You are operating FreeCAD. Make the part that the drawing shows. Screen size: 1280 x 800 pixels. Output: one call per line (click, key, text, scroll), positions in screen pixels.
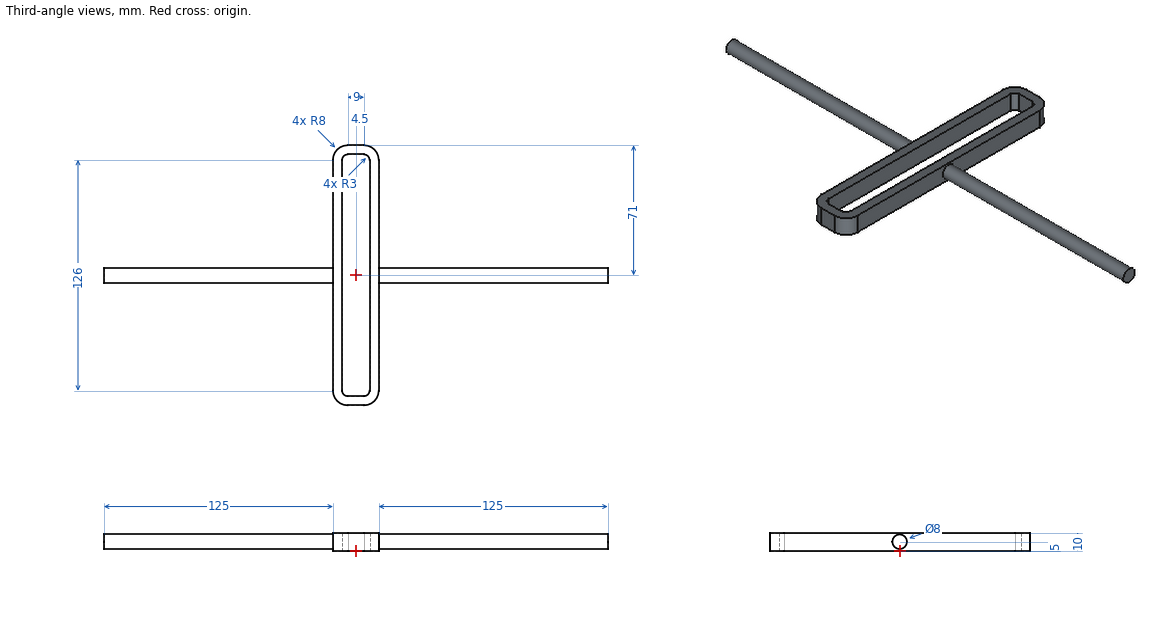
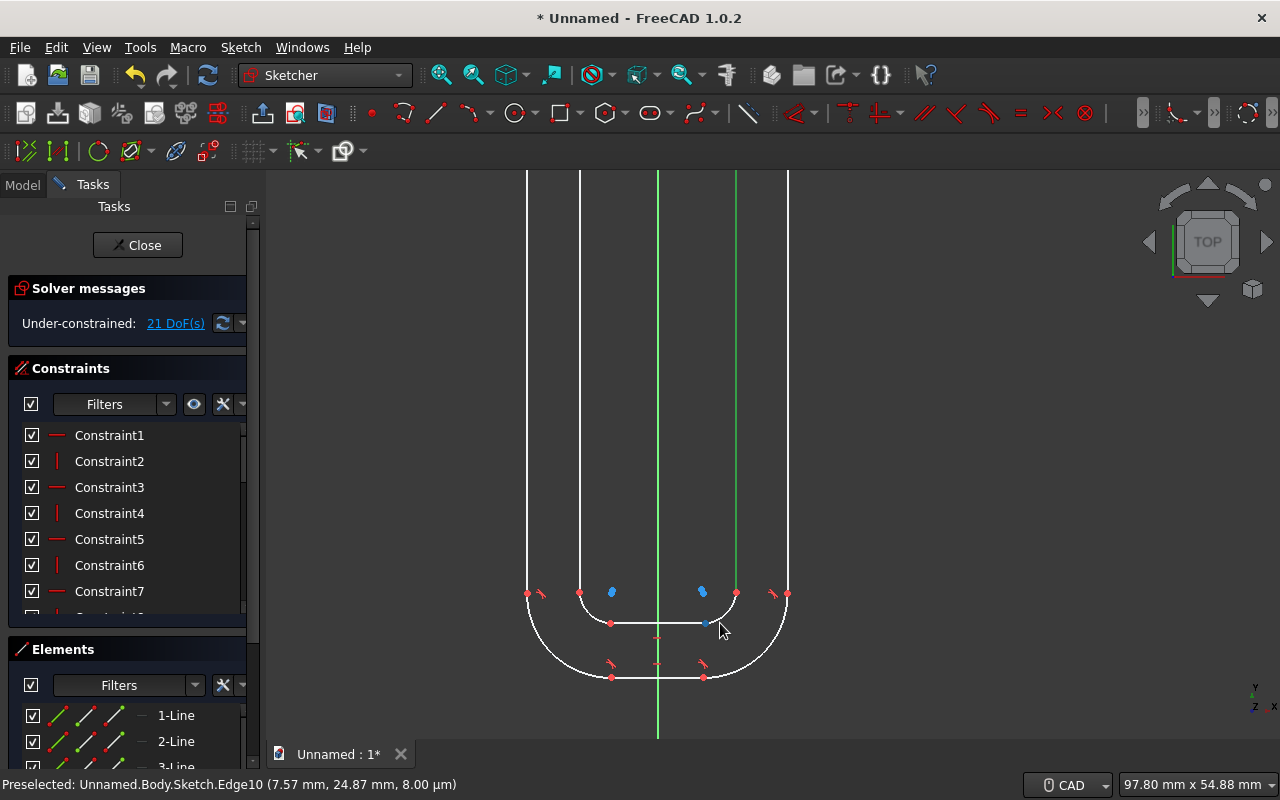
click(719, 619)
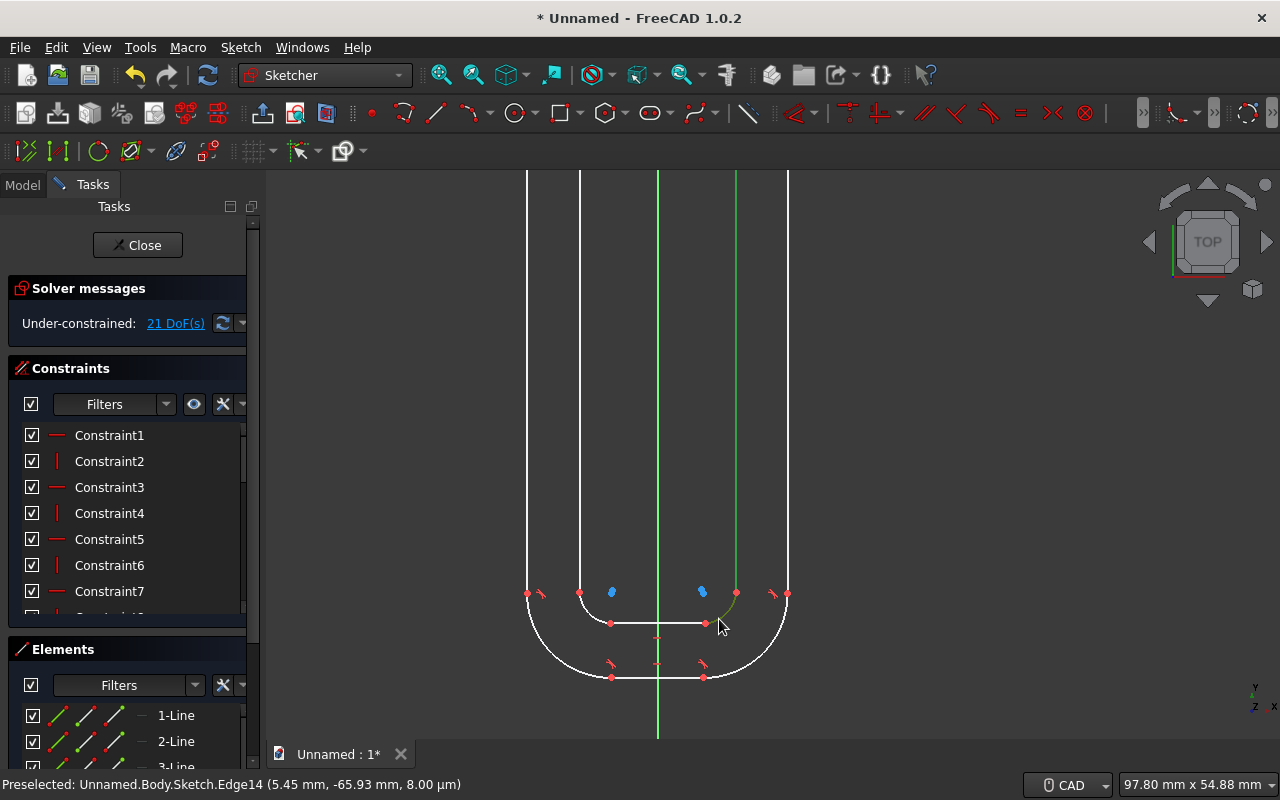
click(990, 114)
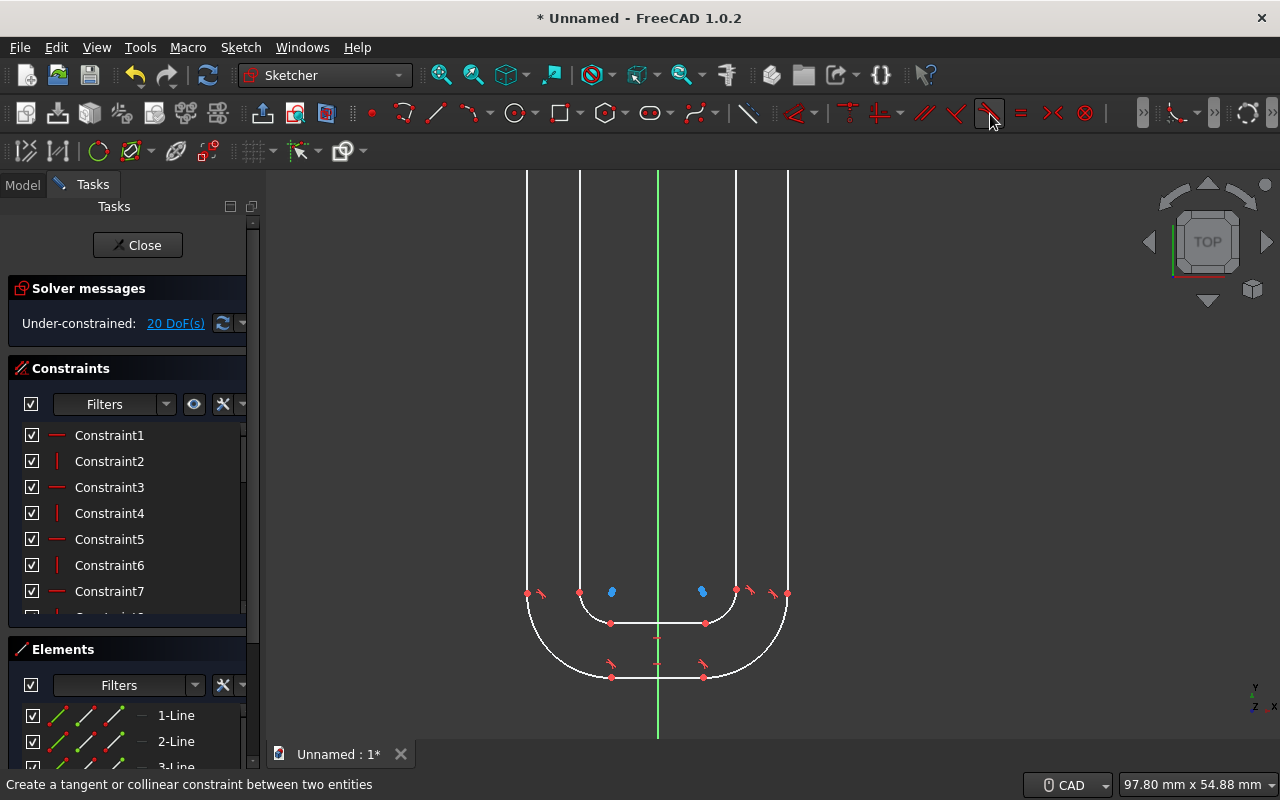
click(677, 623)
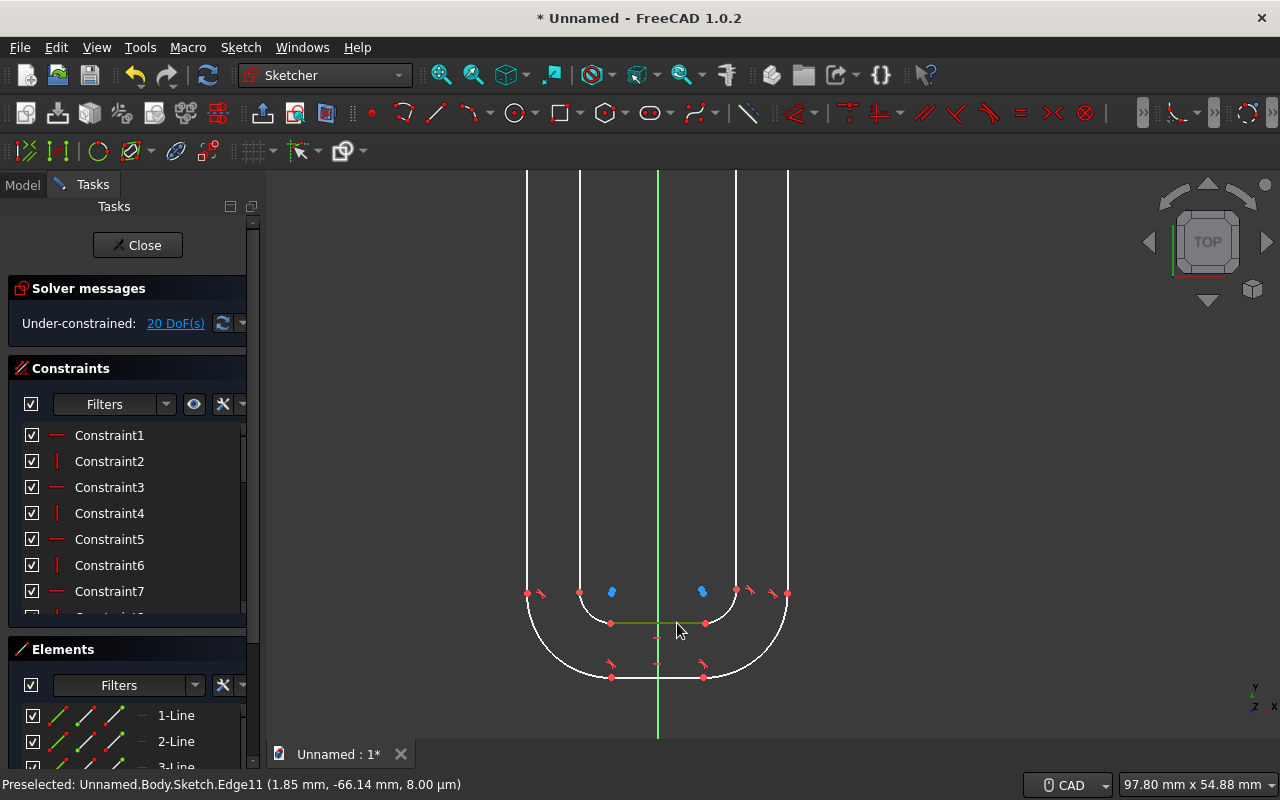
click(719, 619)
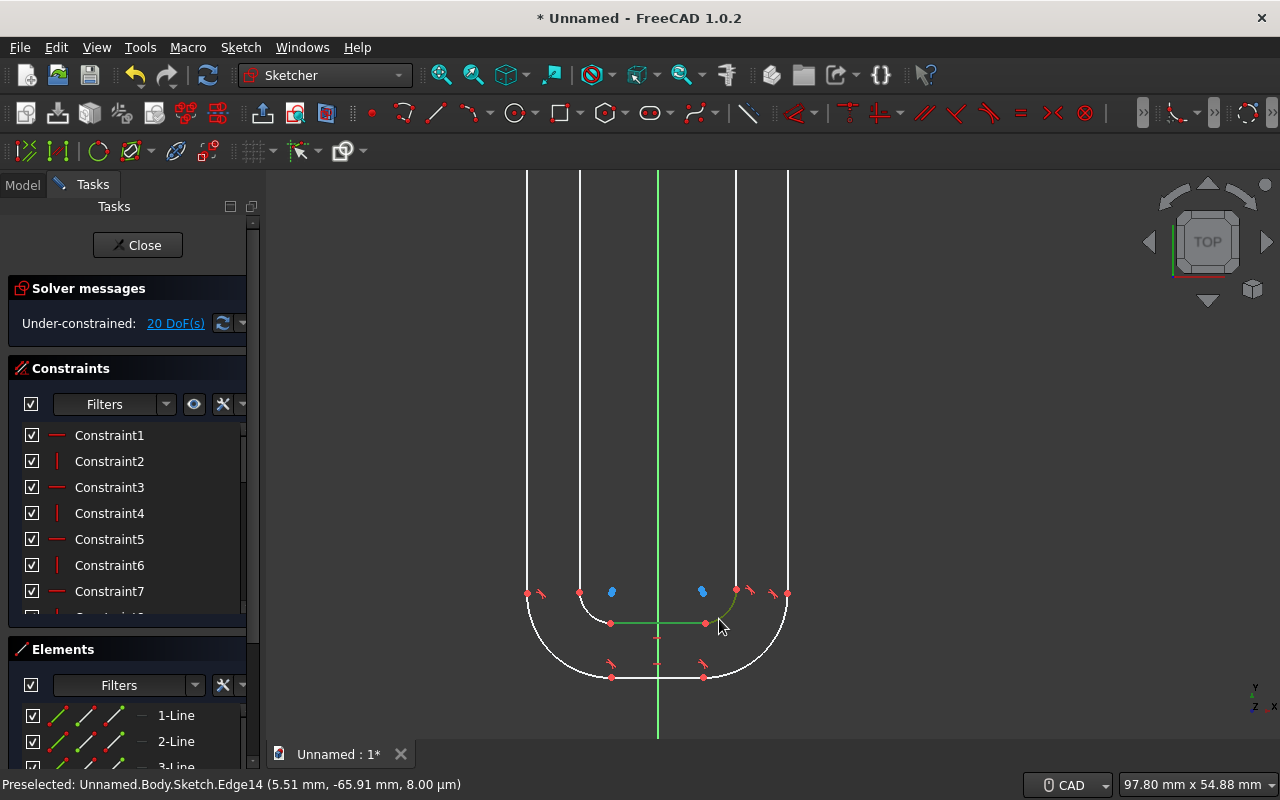
click(990, 114)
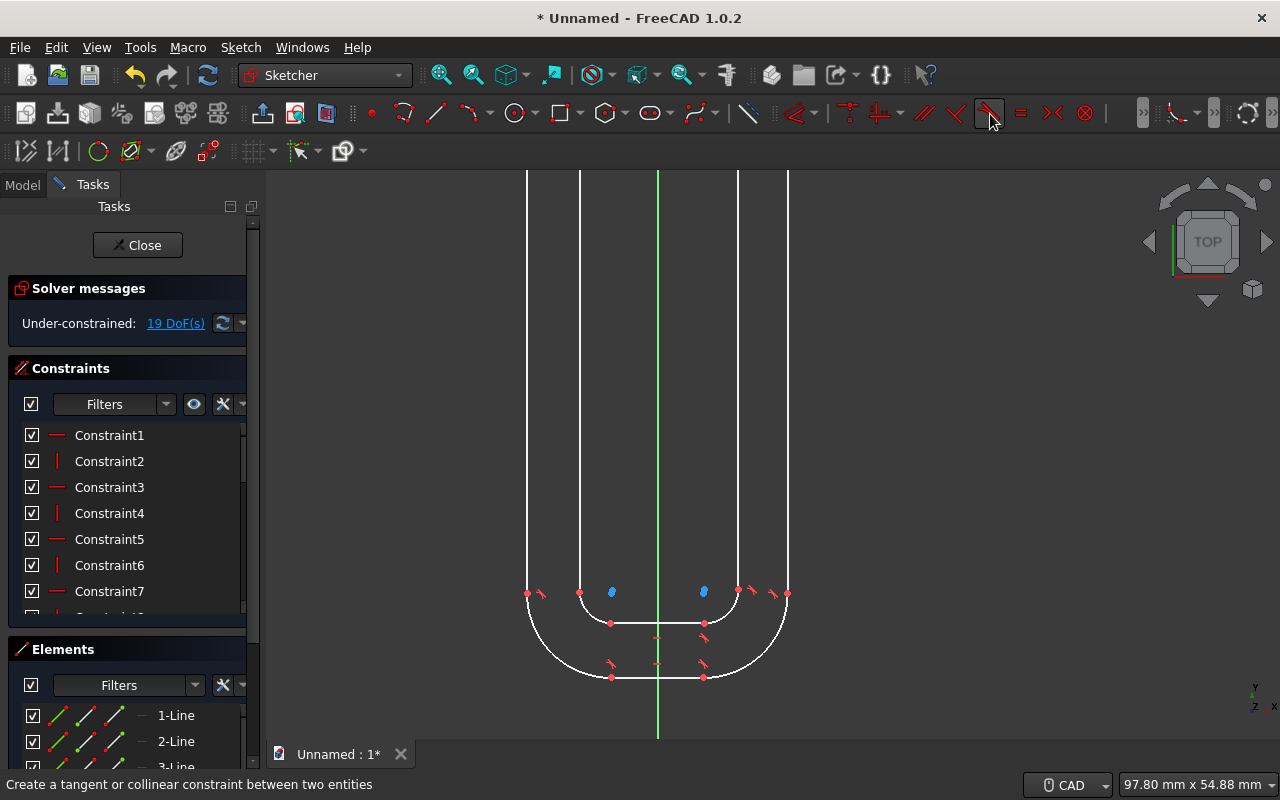
click(676, 623)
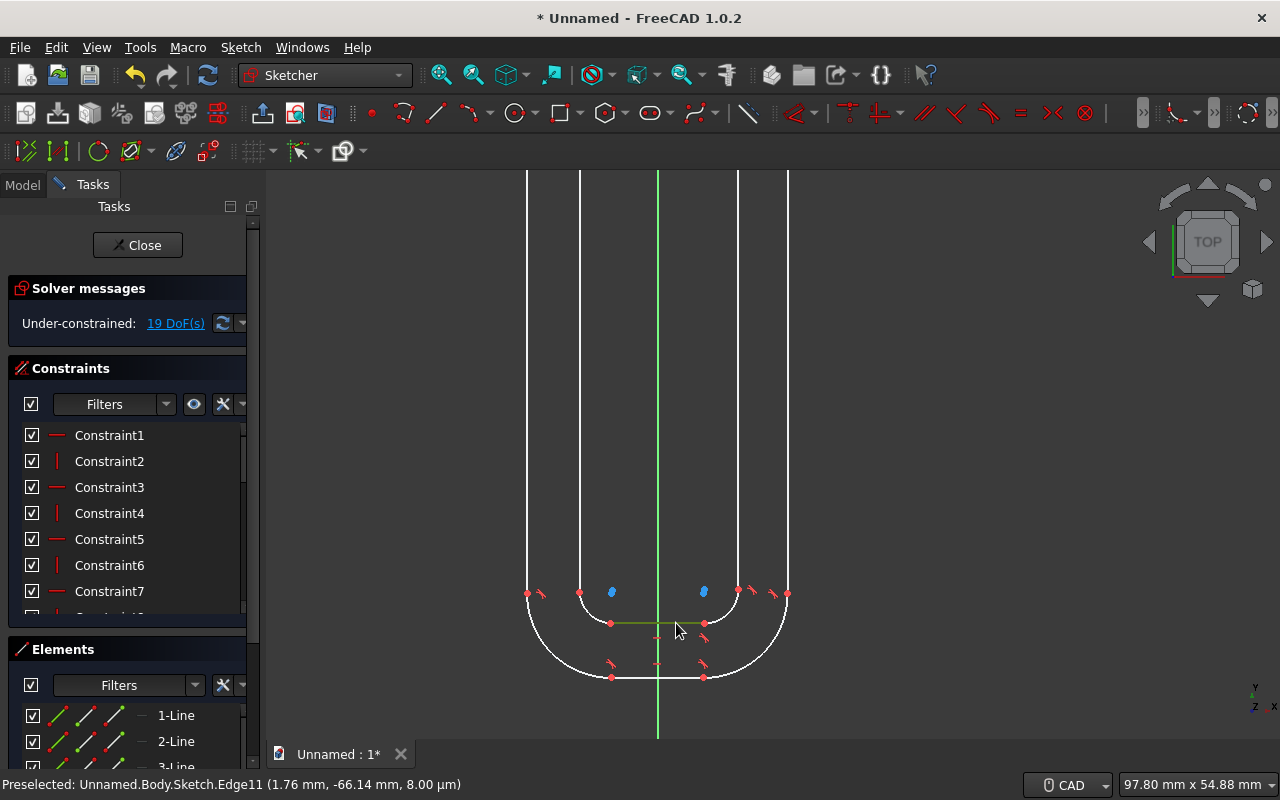
click(584, 606)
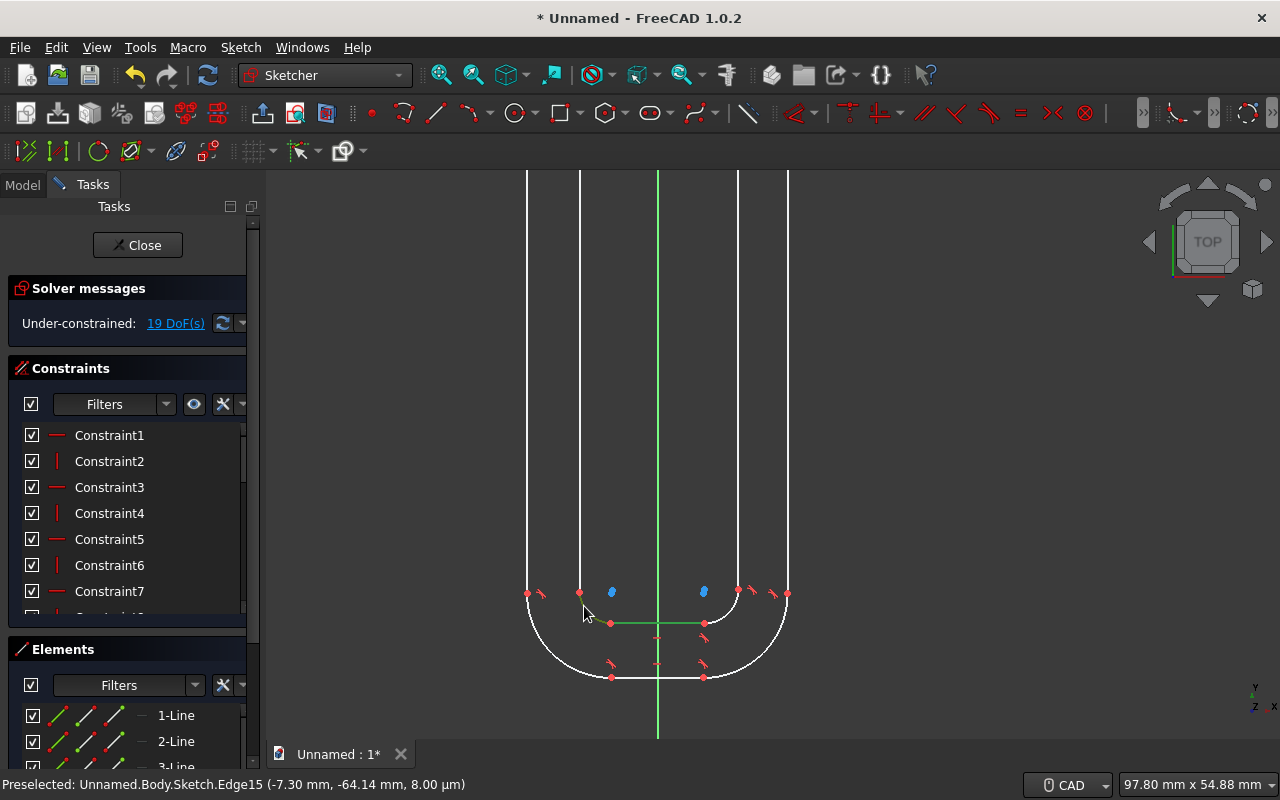
click(990, 114)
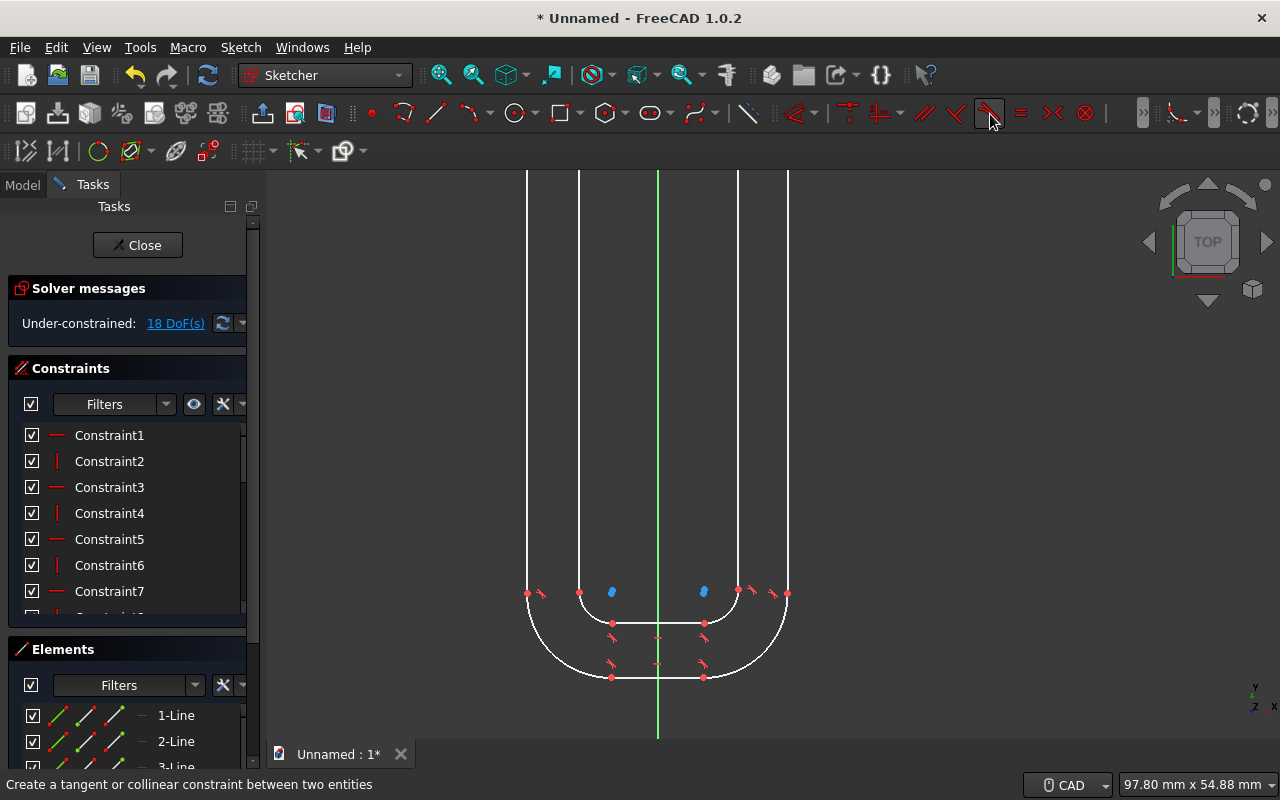
scroll(720, 624, down, 7)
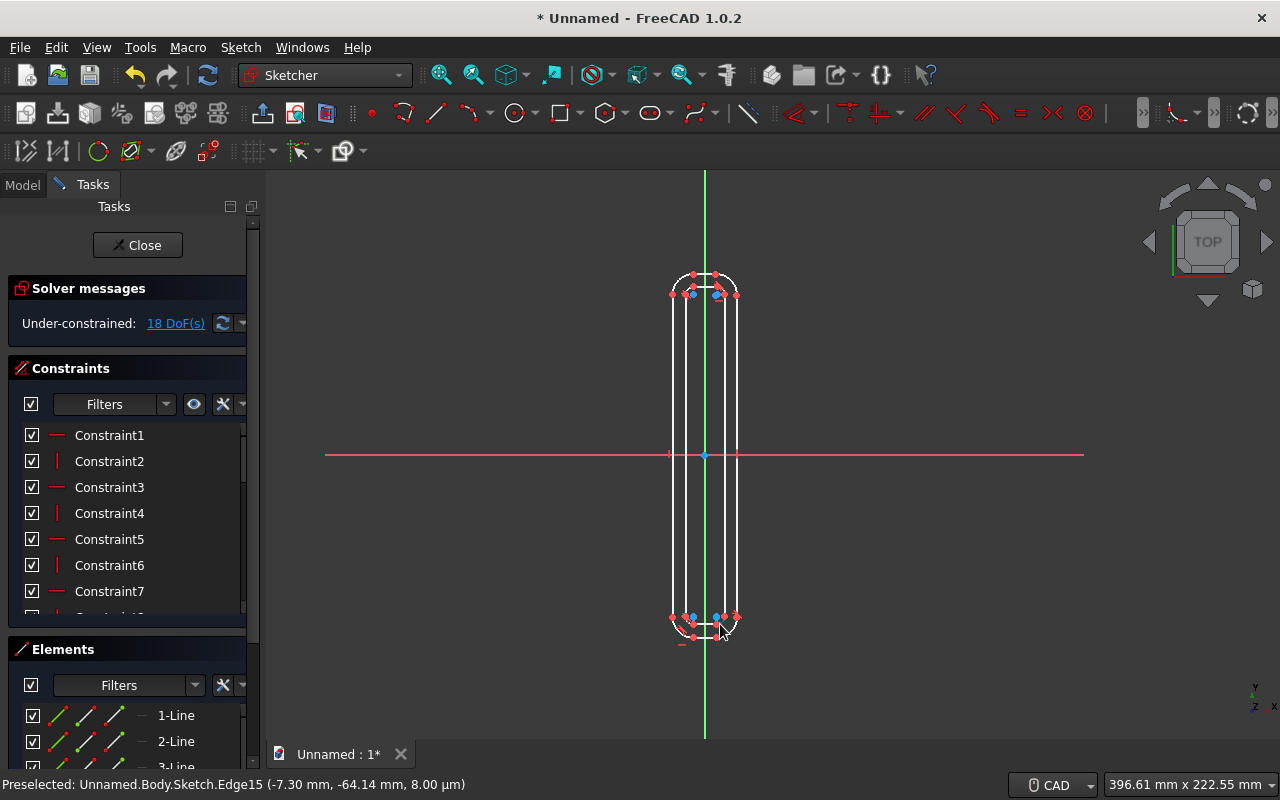
click(686, 520)